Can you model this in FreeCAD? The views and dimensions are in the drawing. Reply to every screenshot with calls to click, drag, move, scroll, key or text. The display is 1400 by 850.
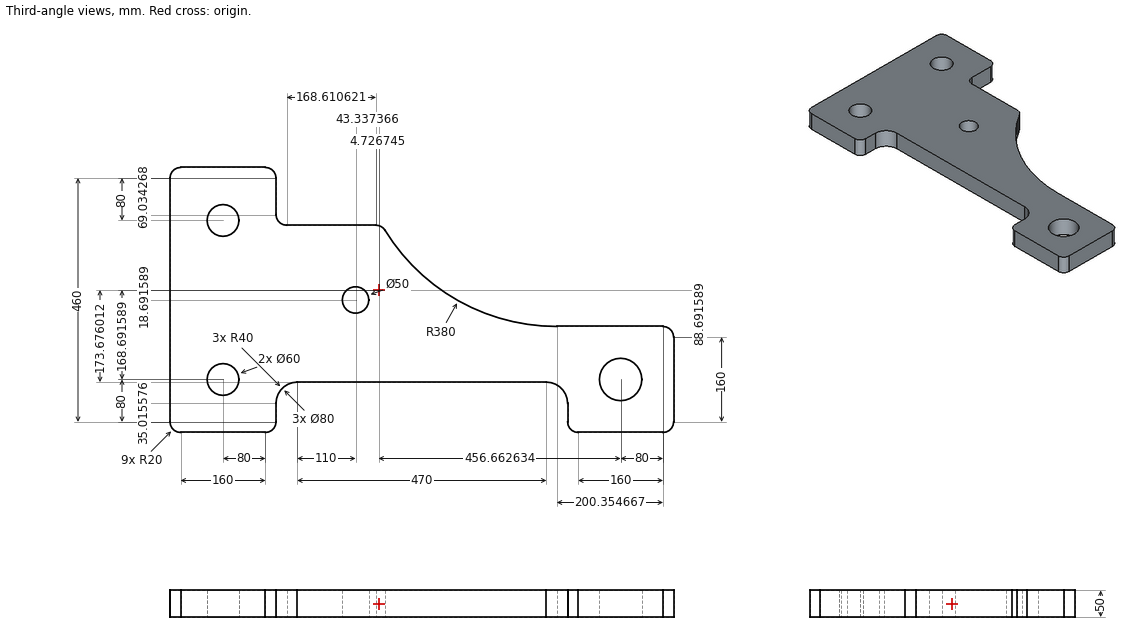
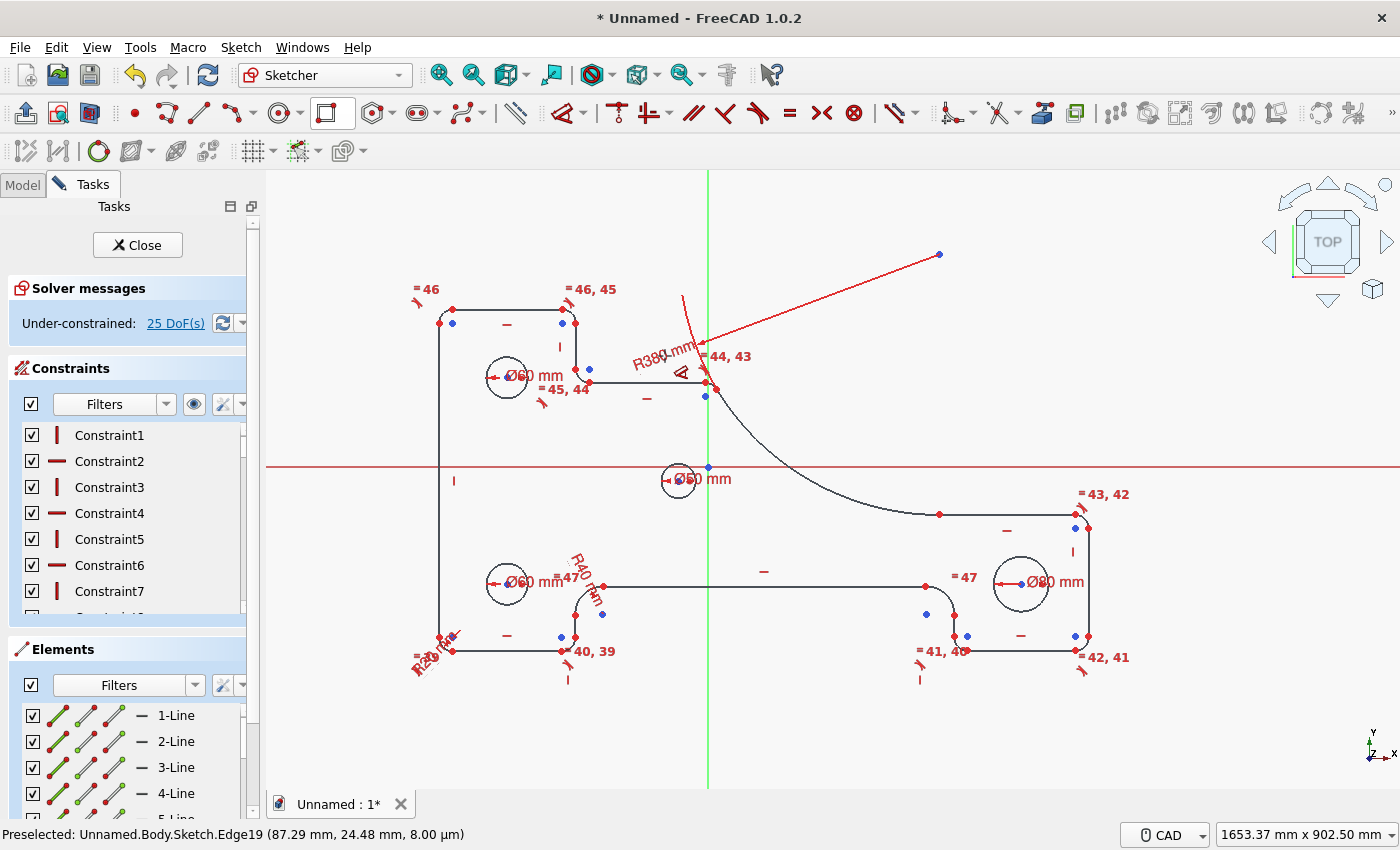
click(439, 418)
click(405, 480)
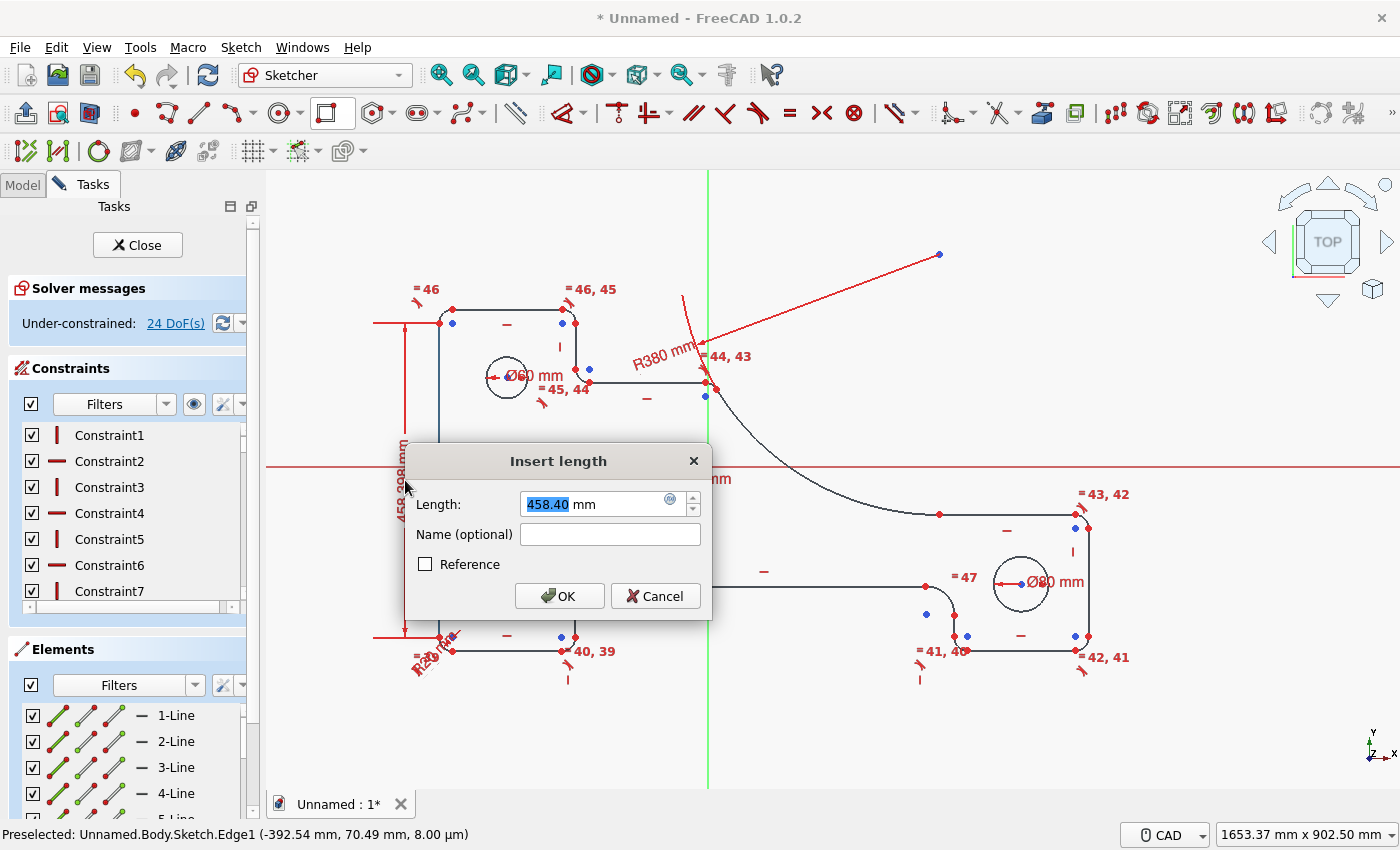
text(460)
key(Return)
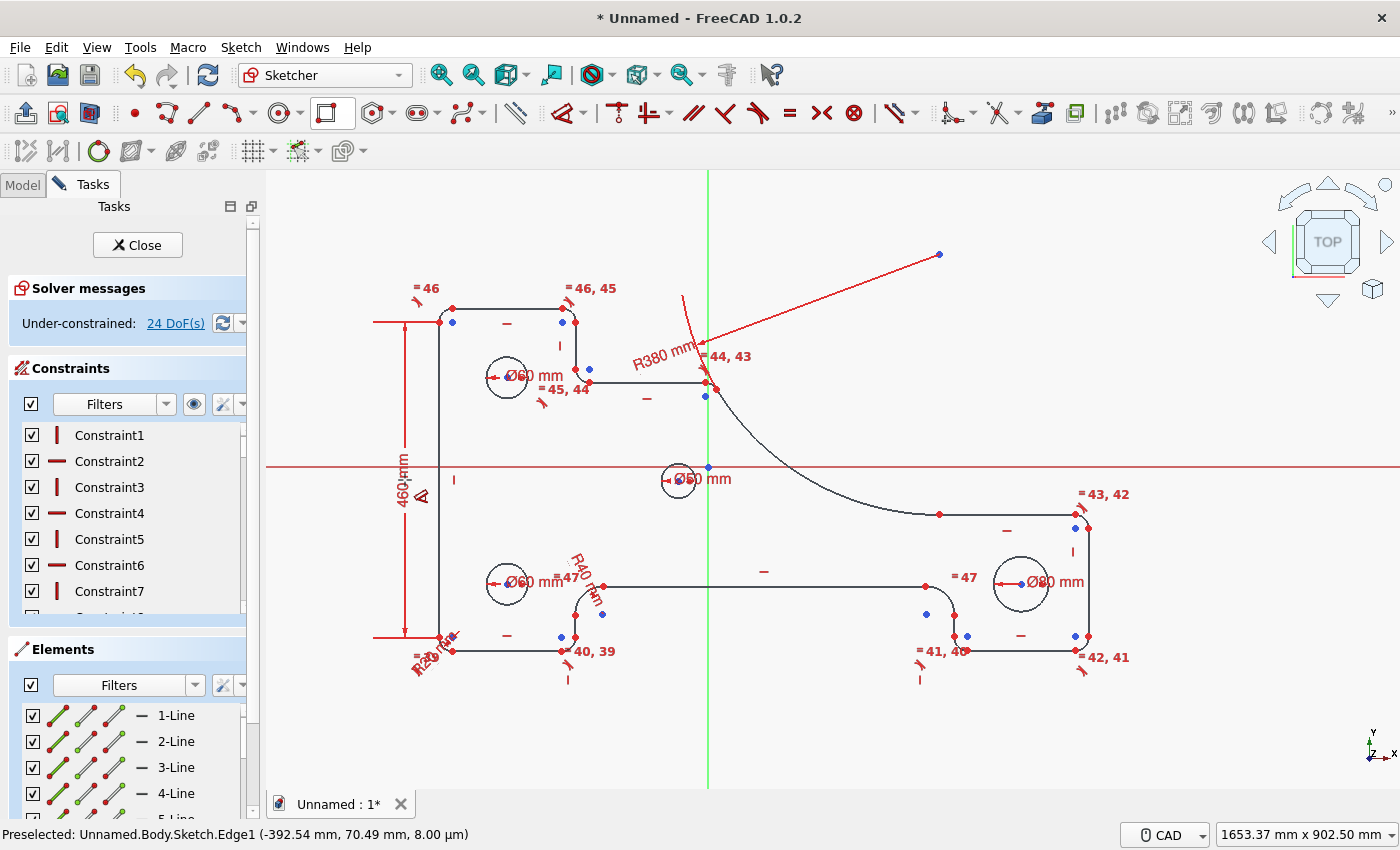
click(486, 651)
click(507, 685)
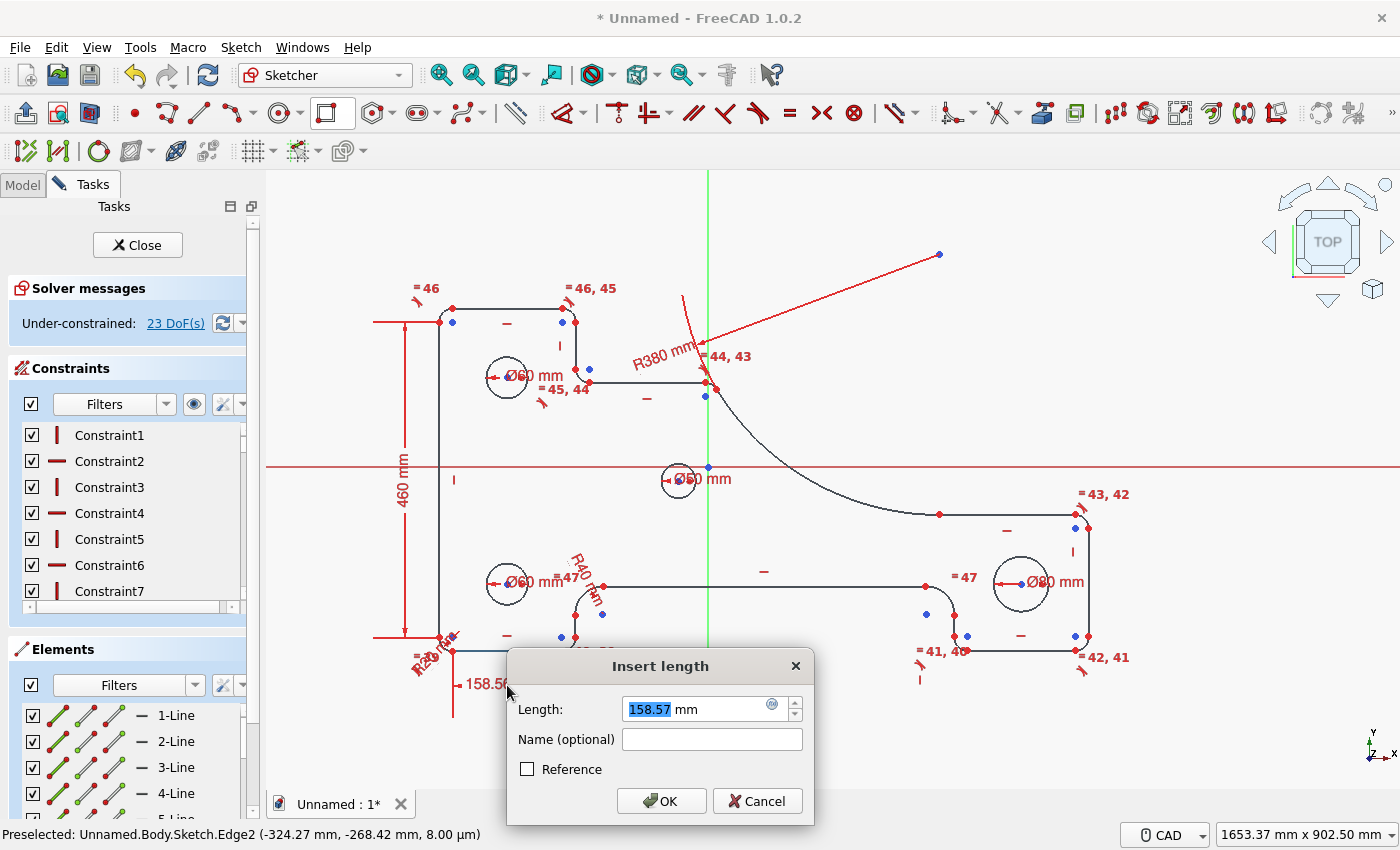
text(160)
key(Return)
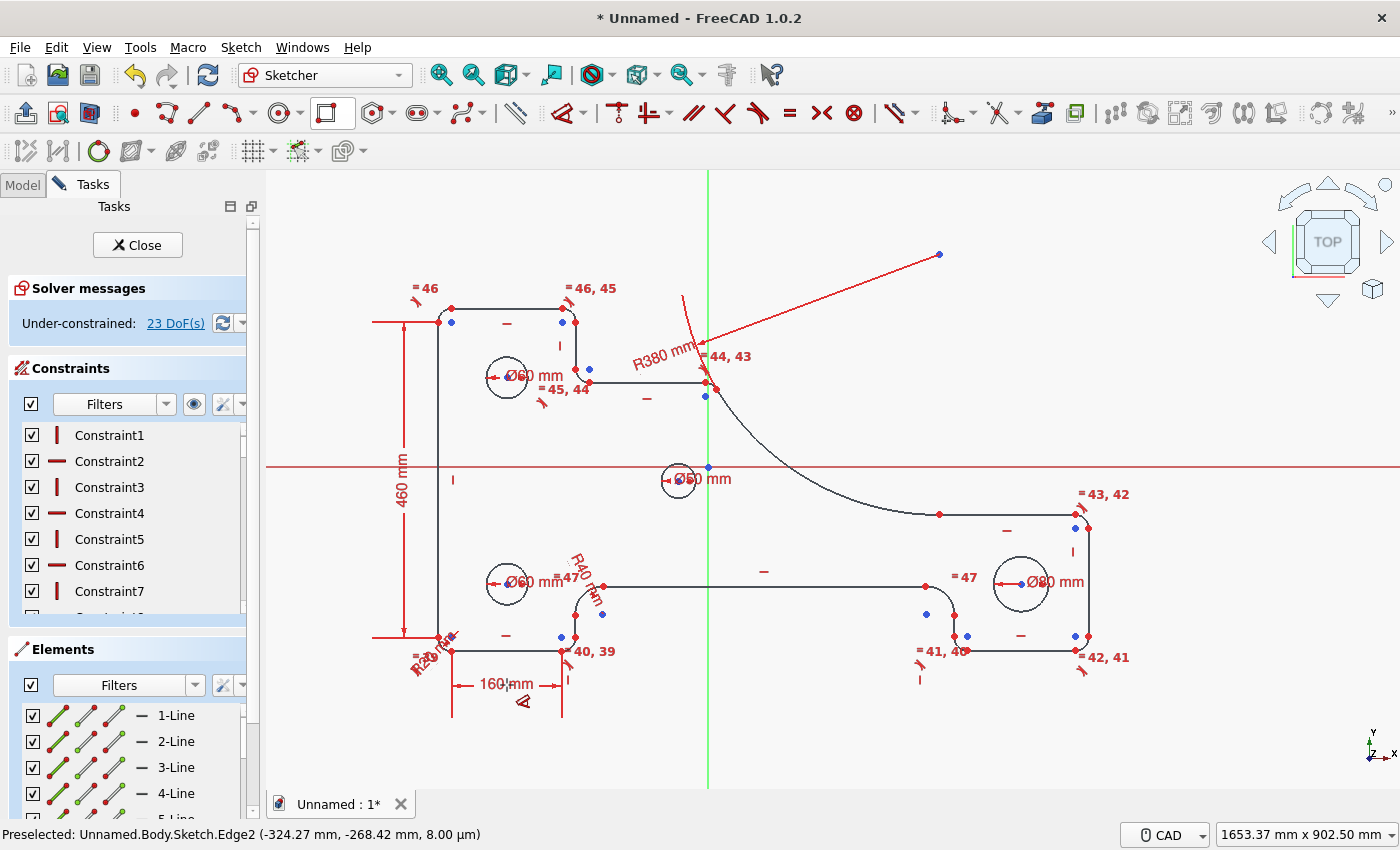
click(829, 587)
click(765, 621)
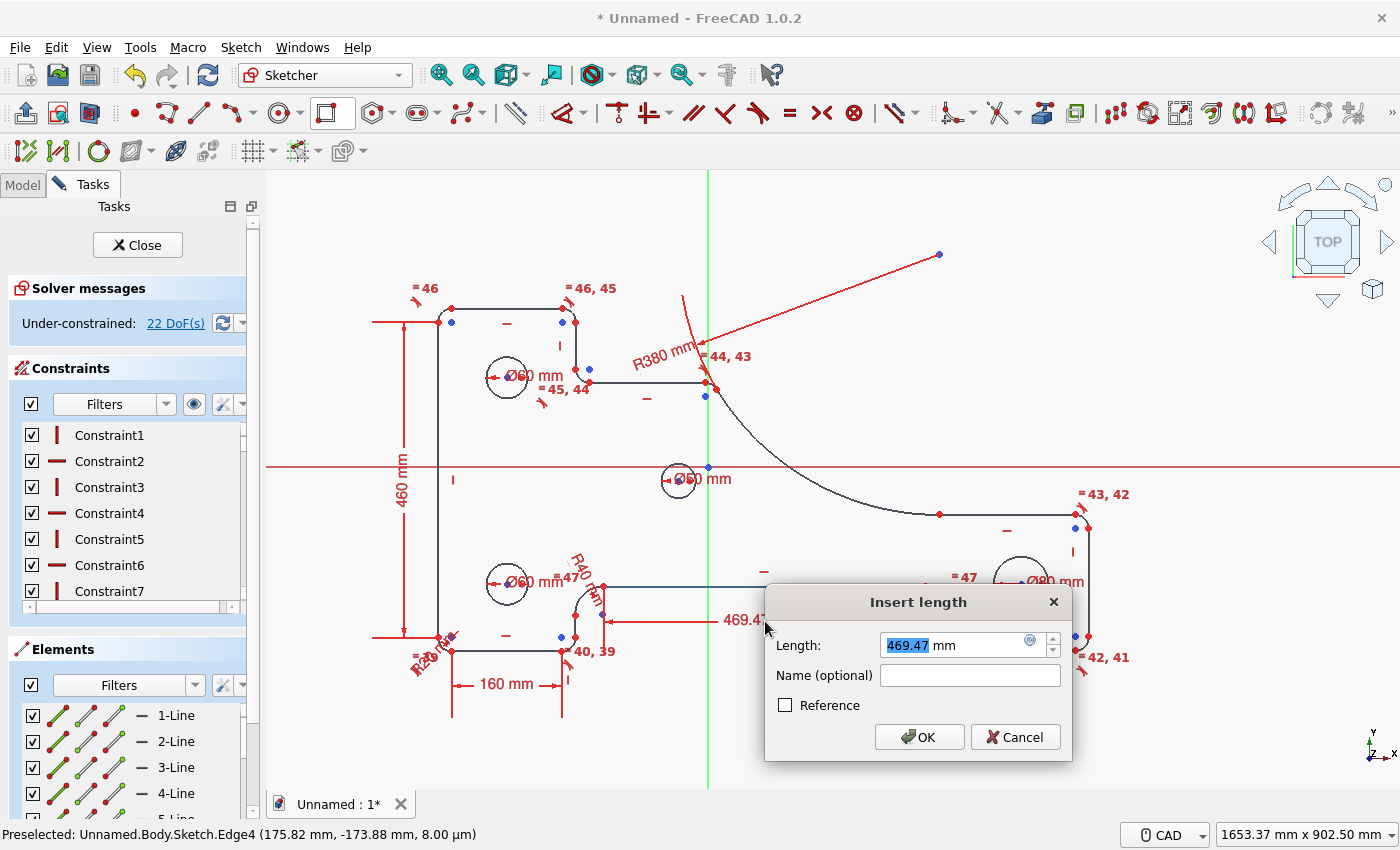
text(470)
key(Return)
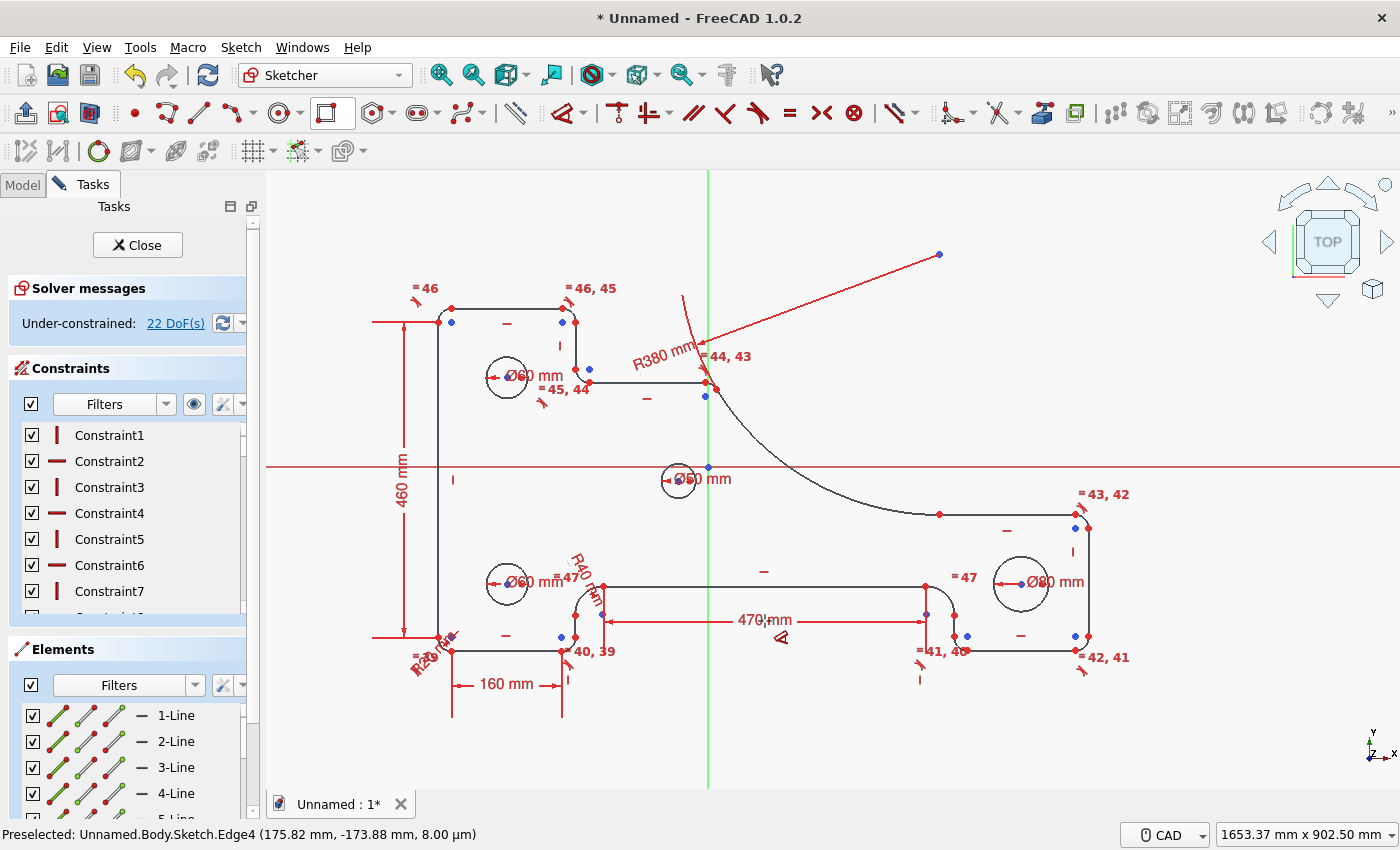
click(1000, 651)
click(1022, 685)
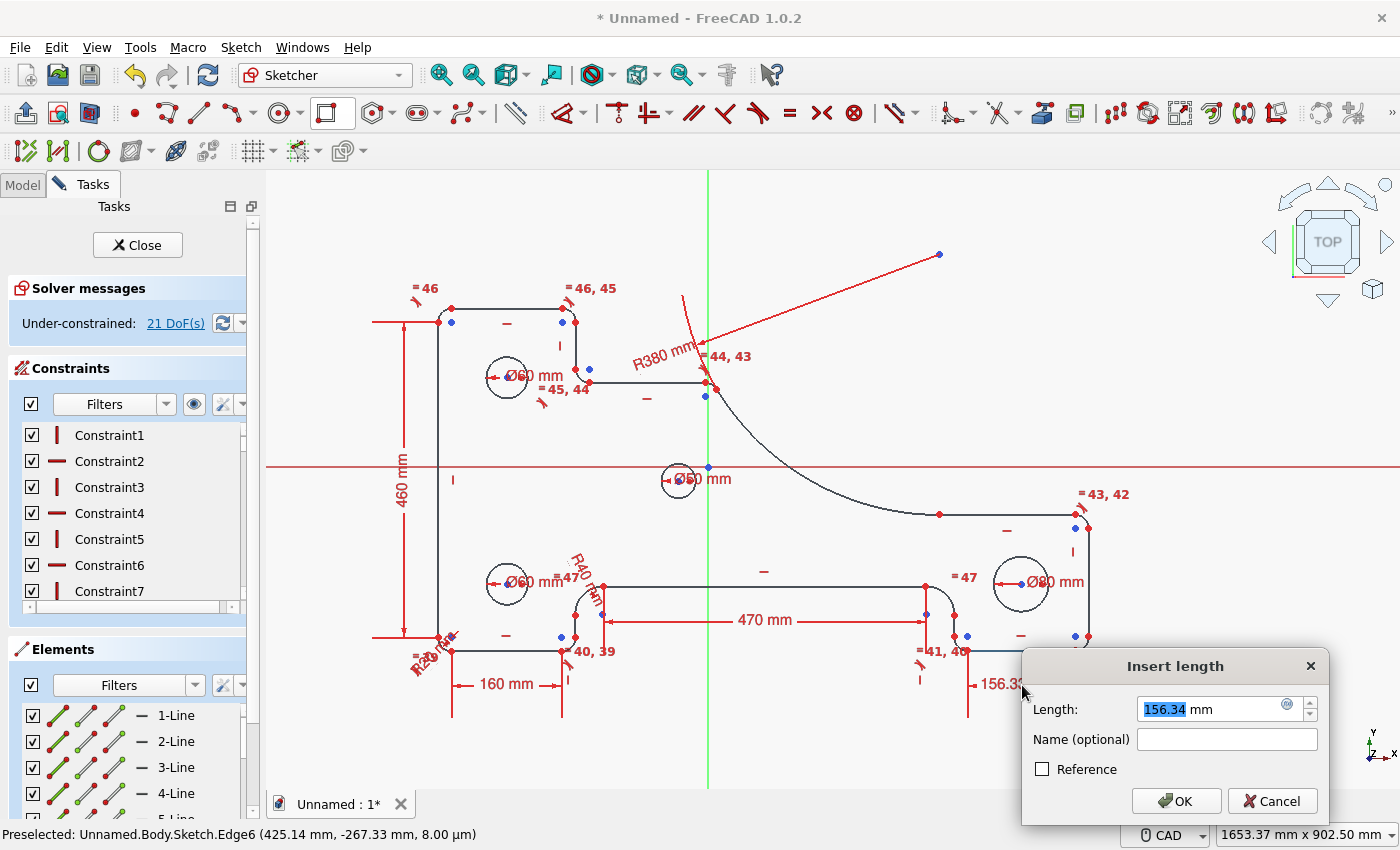
text(160)
key(Return)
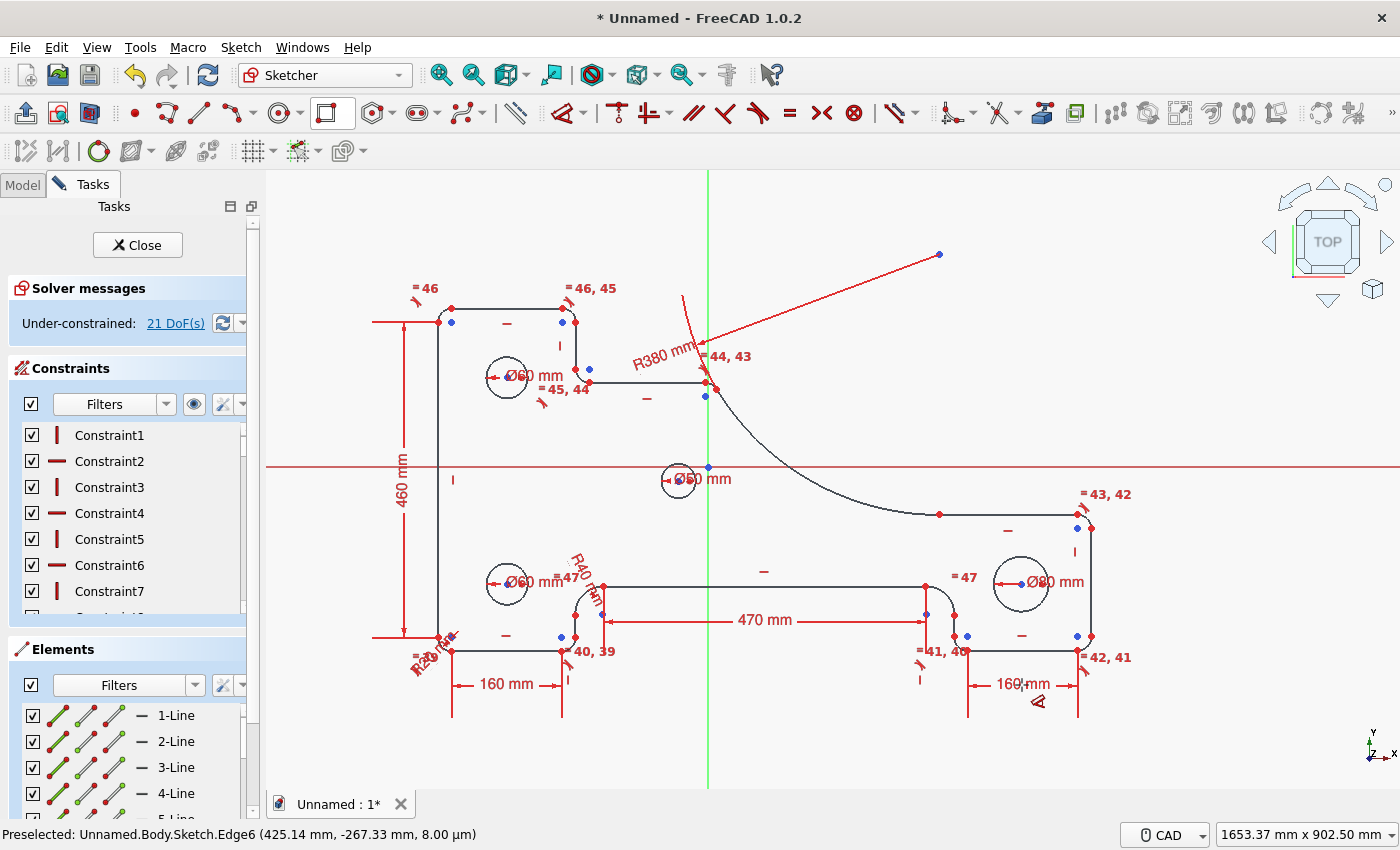
click(1091, 604)
click(1125, 583)